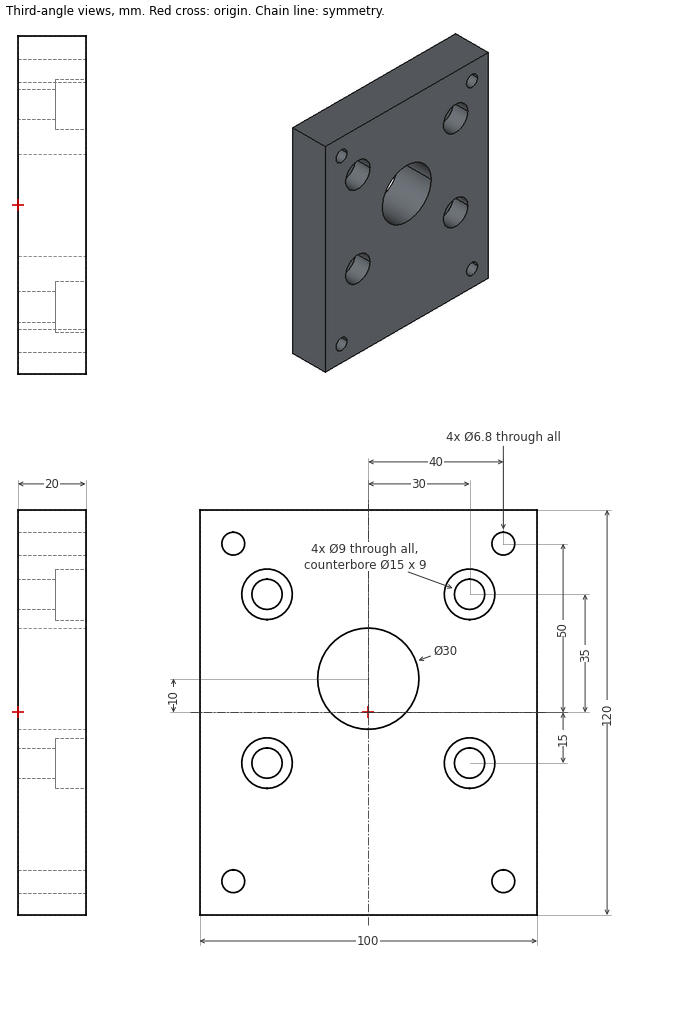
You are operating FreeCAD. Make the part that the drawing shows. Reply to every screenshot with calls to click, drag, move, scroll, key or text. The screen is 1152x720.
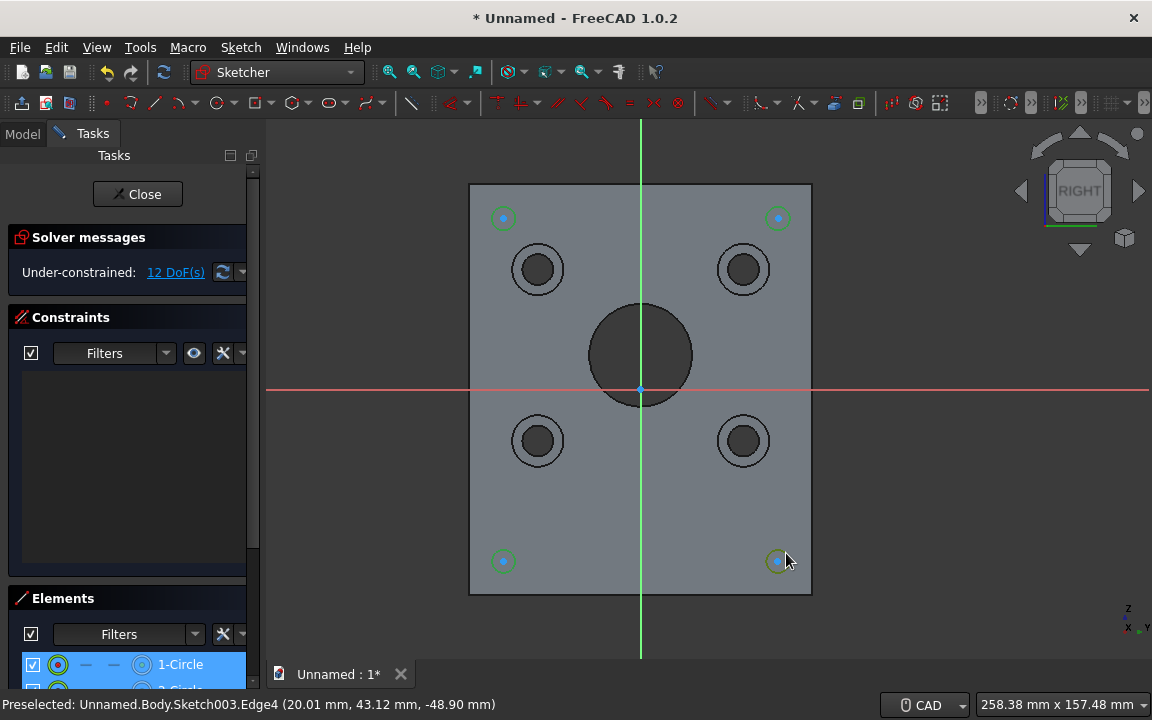
click(630, 104)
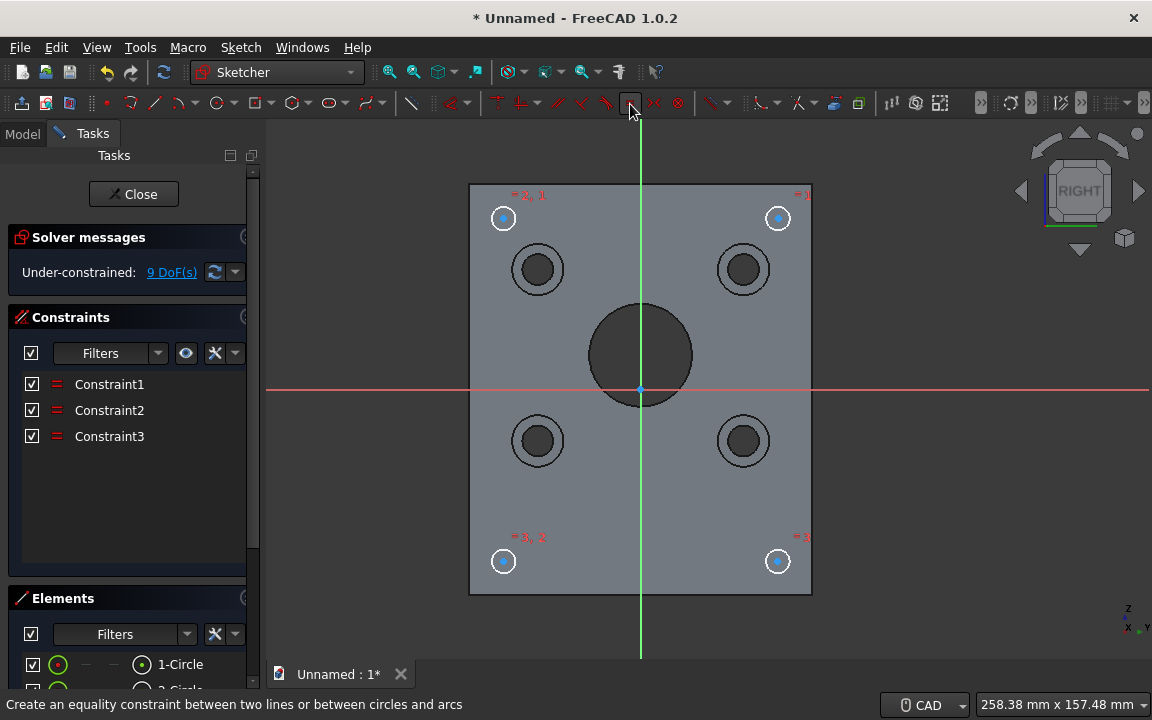
click(778, 219)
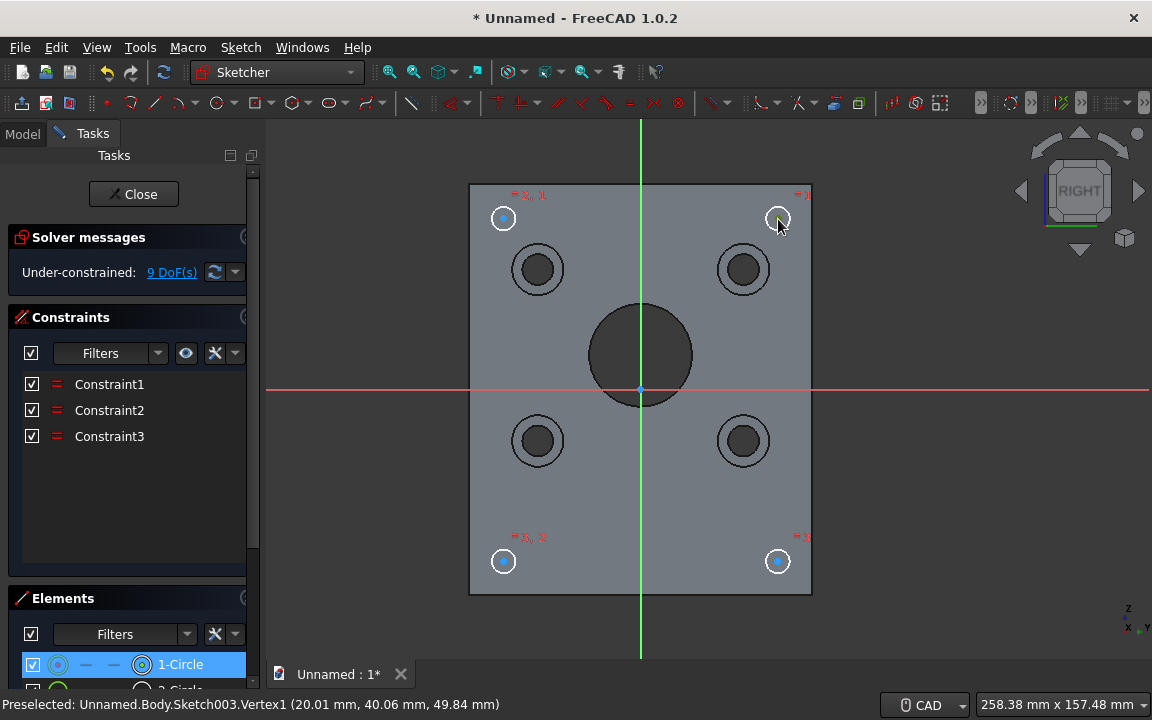
click(504, 219)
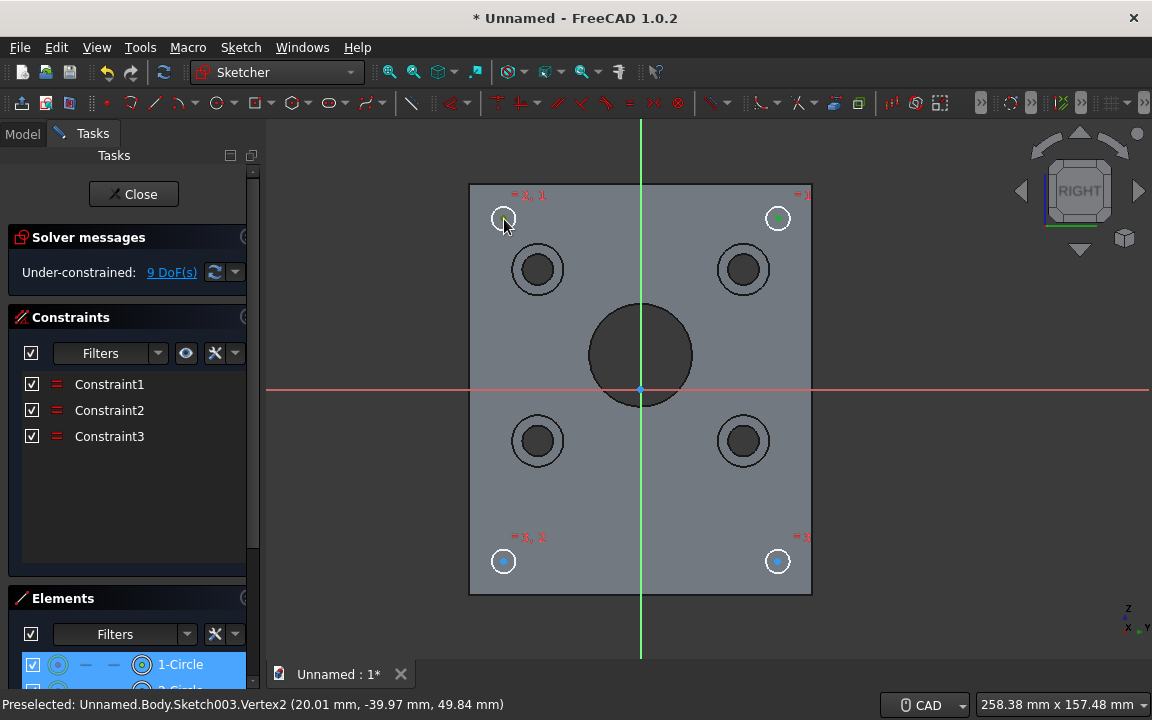
click(641, 596)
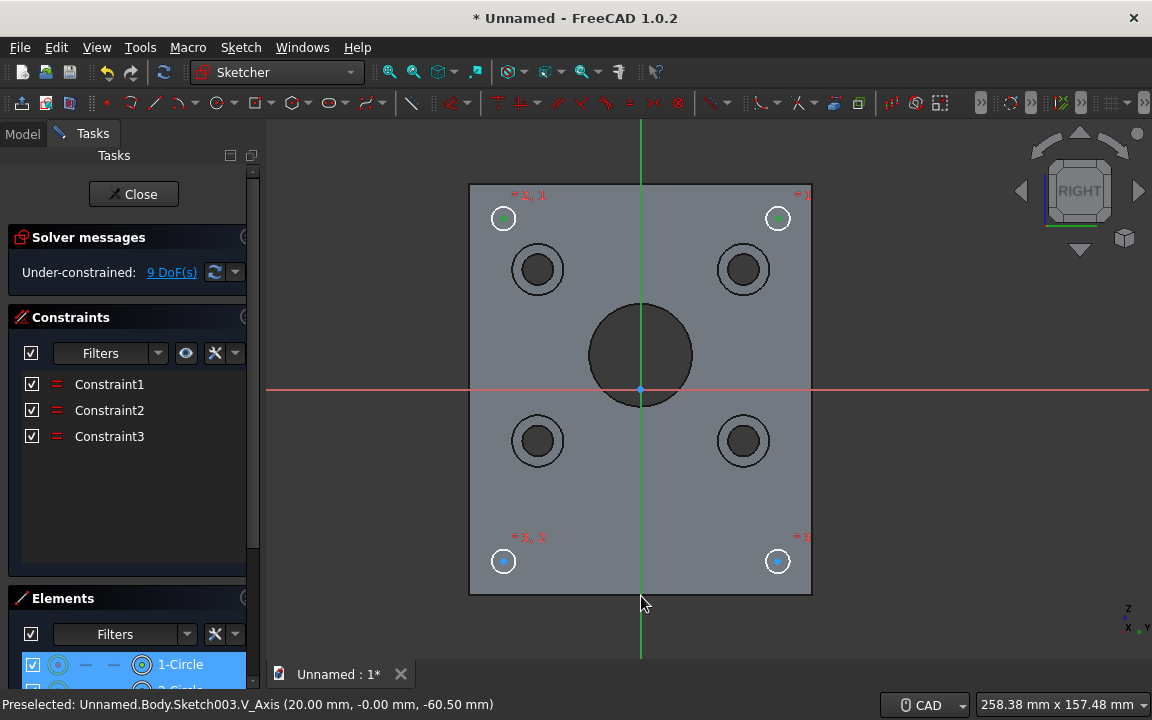
click(654, 104)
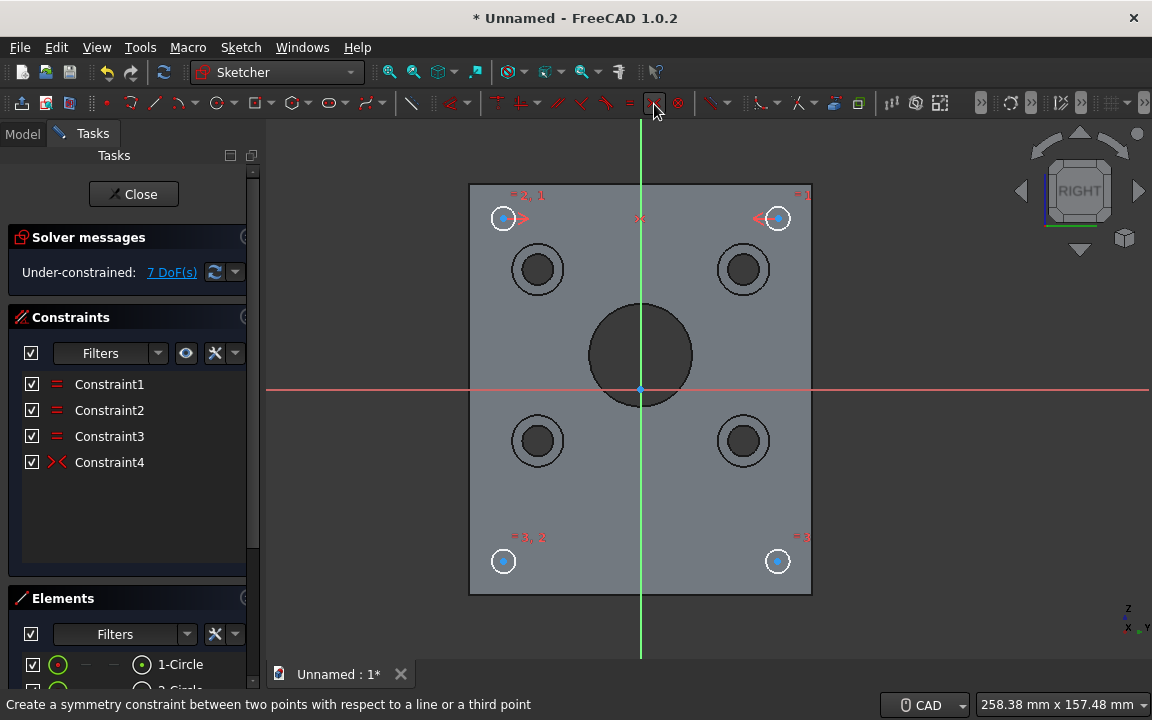
click(503, 219)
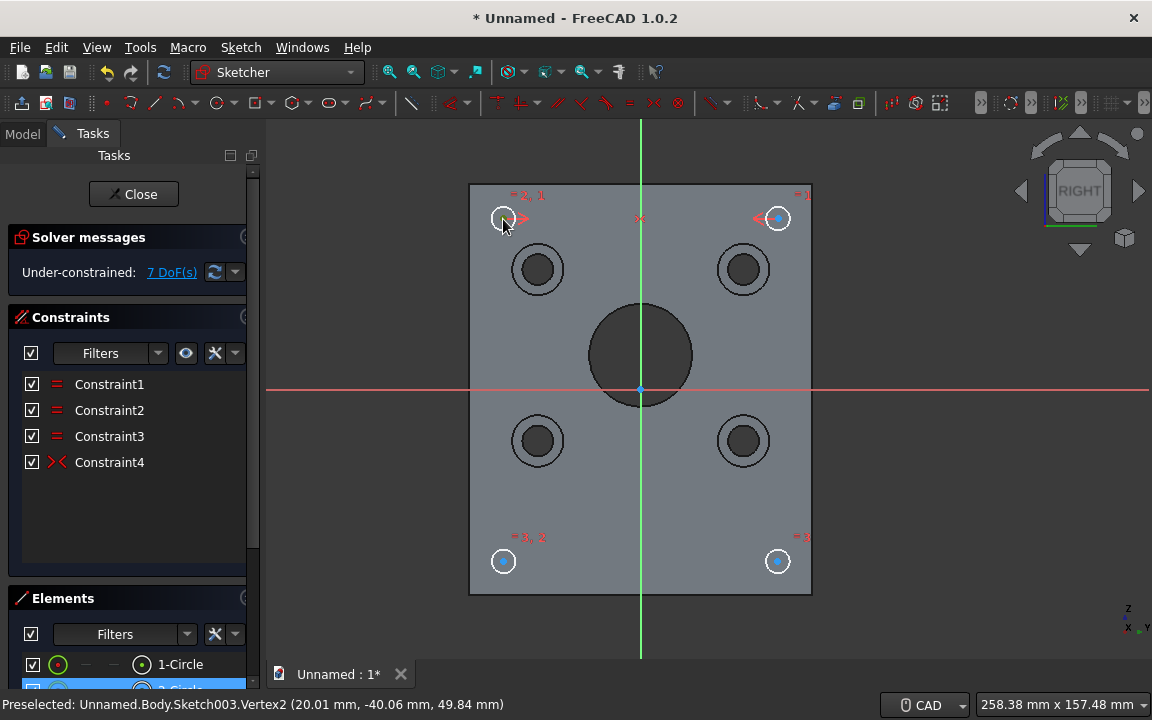
click(504, 561)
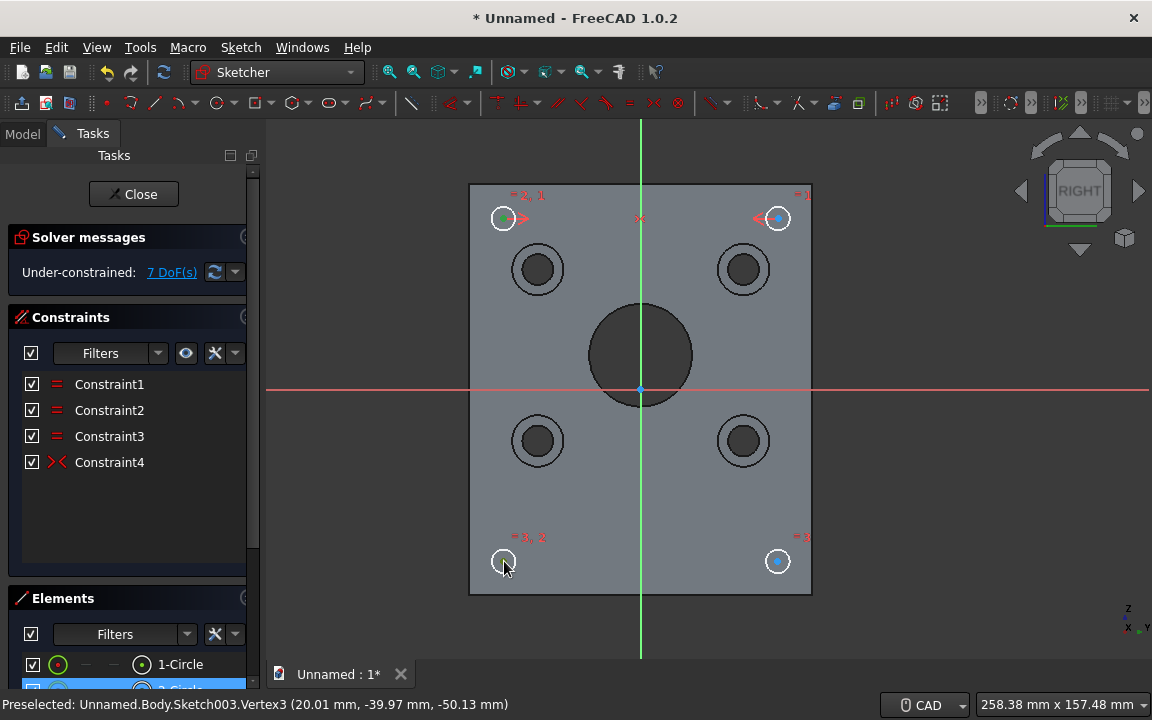
click(344, 390)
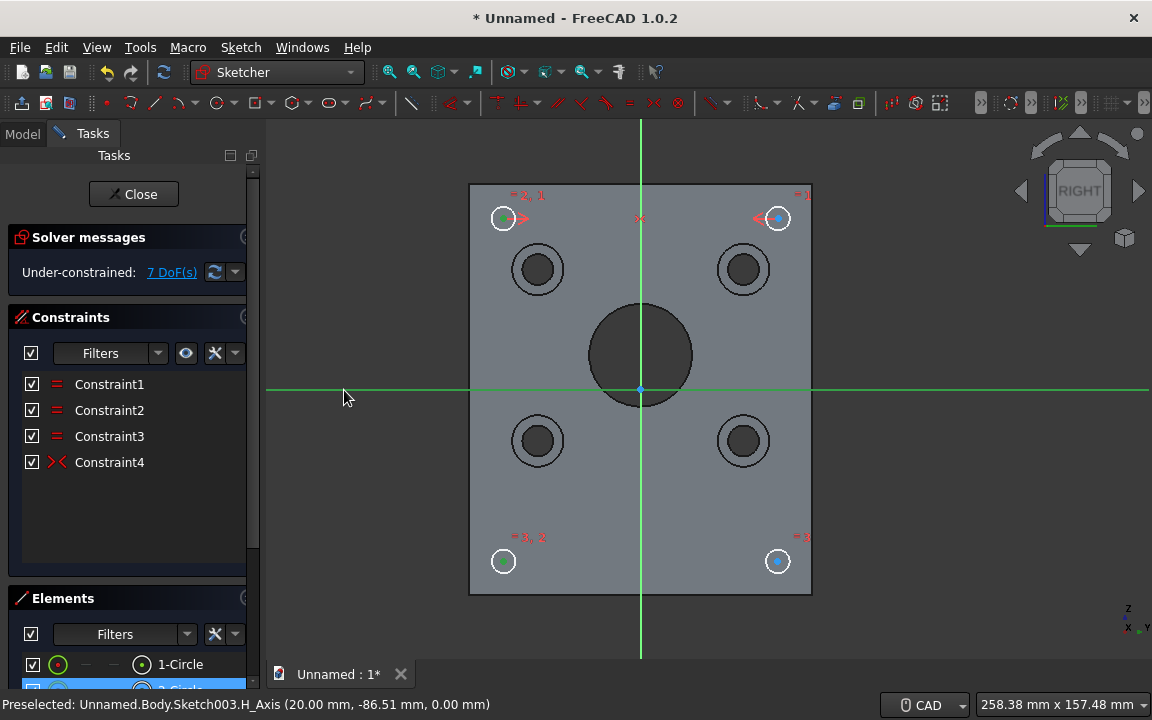
click(654, 104)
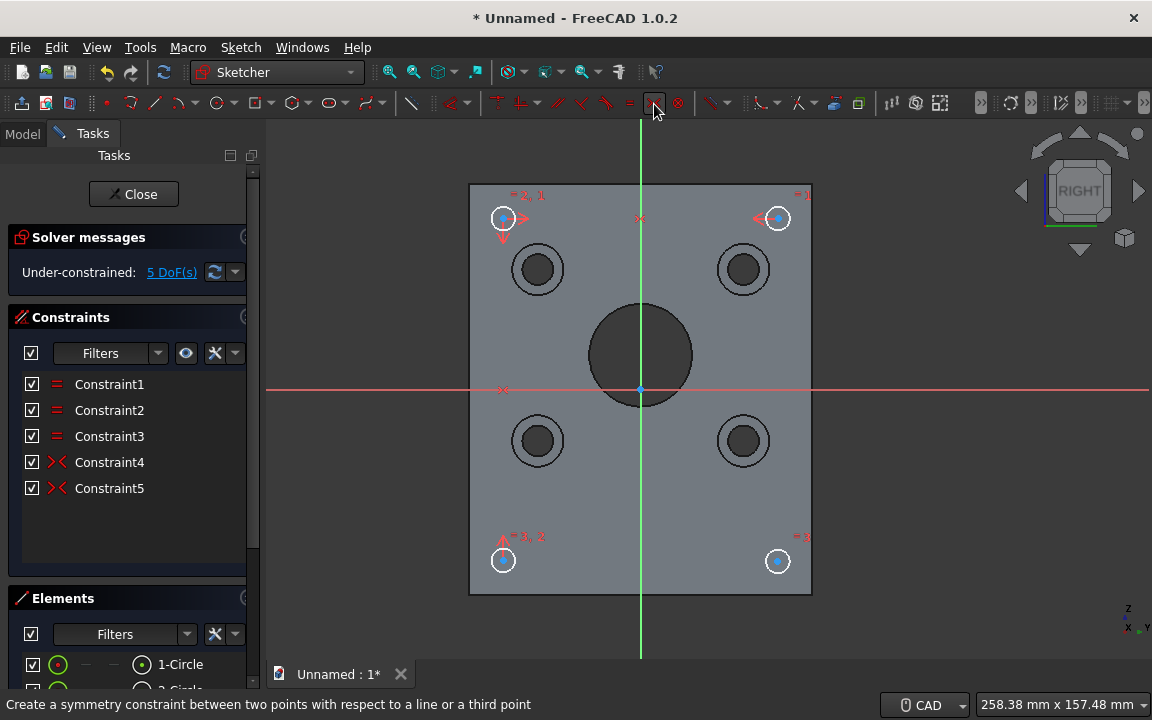
click(778, 219)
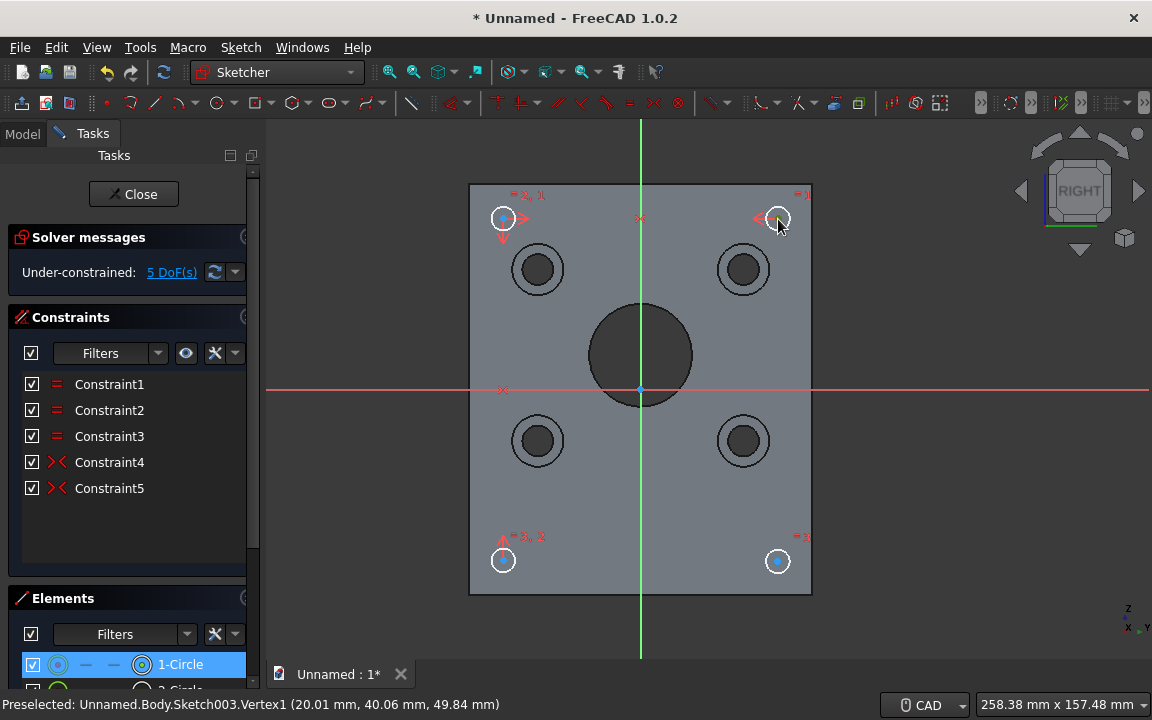
click(778, 561)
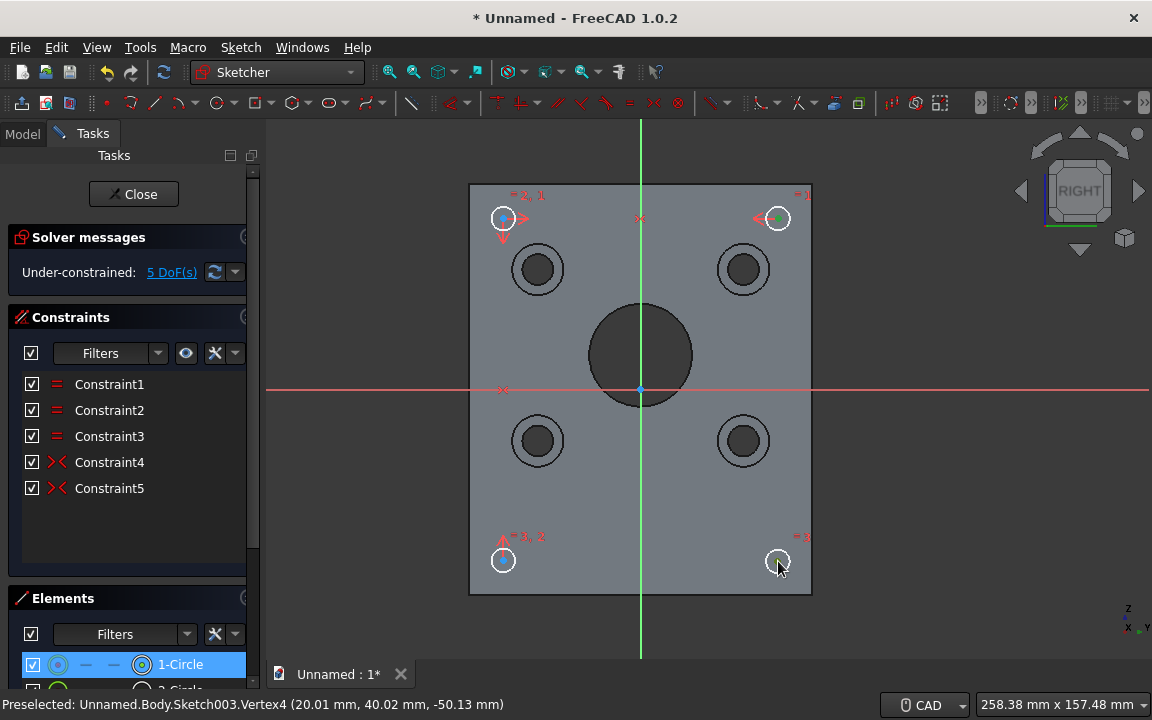
click(344, 390)